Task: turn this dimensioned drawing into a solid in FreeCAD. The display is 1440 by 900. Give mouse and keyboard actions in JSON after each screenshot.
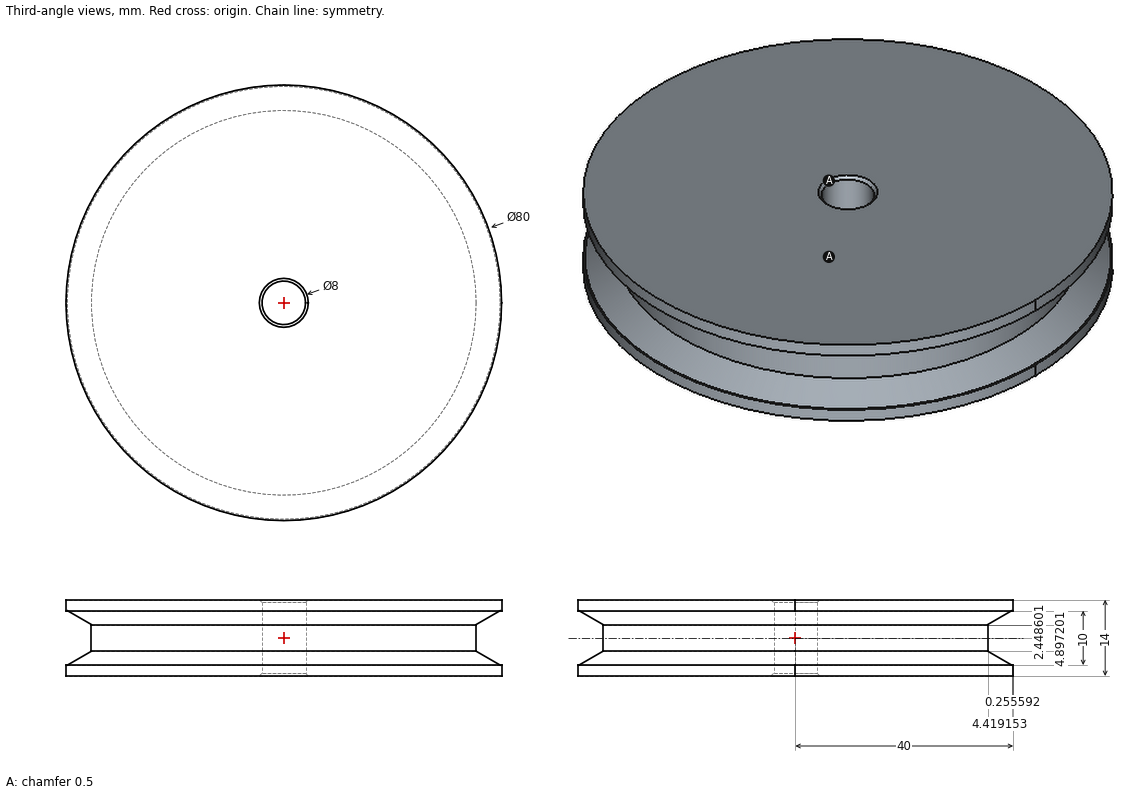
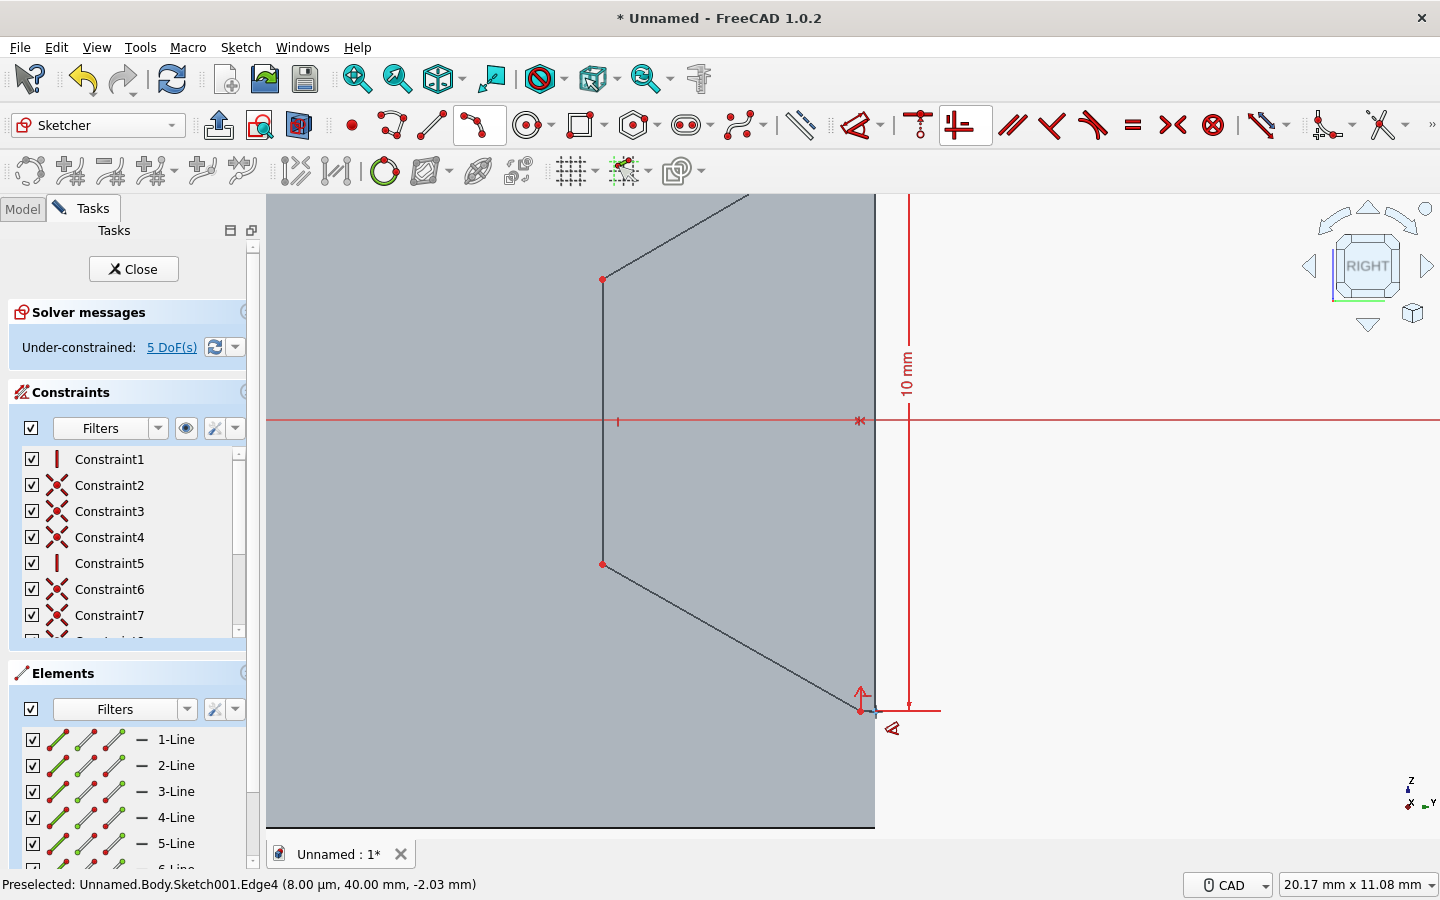
{"action": "left_click", "coordinate": [875, 711]}
{"action": "left_click", "coordinate": [585, 745]}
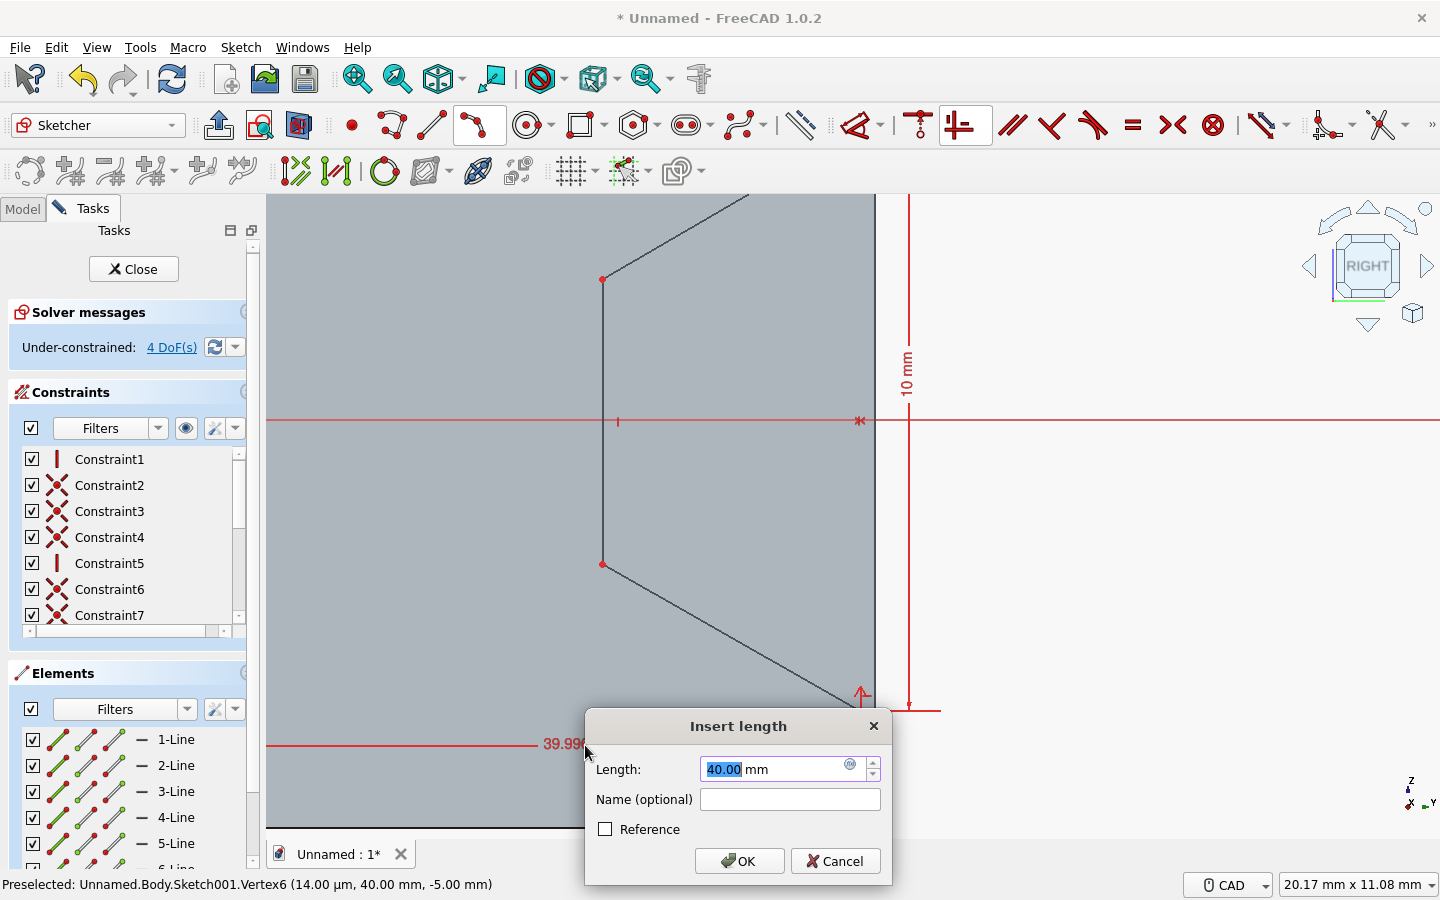
{"action": "type", "text": "40"}
{"action": "key", "text": "Return"}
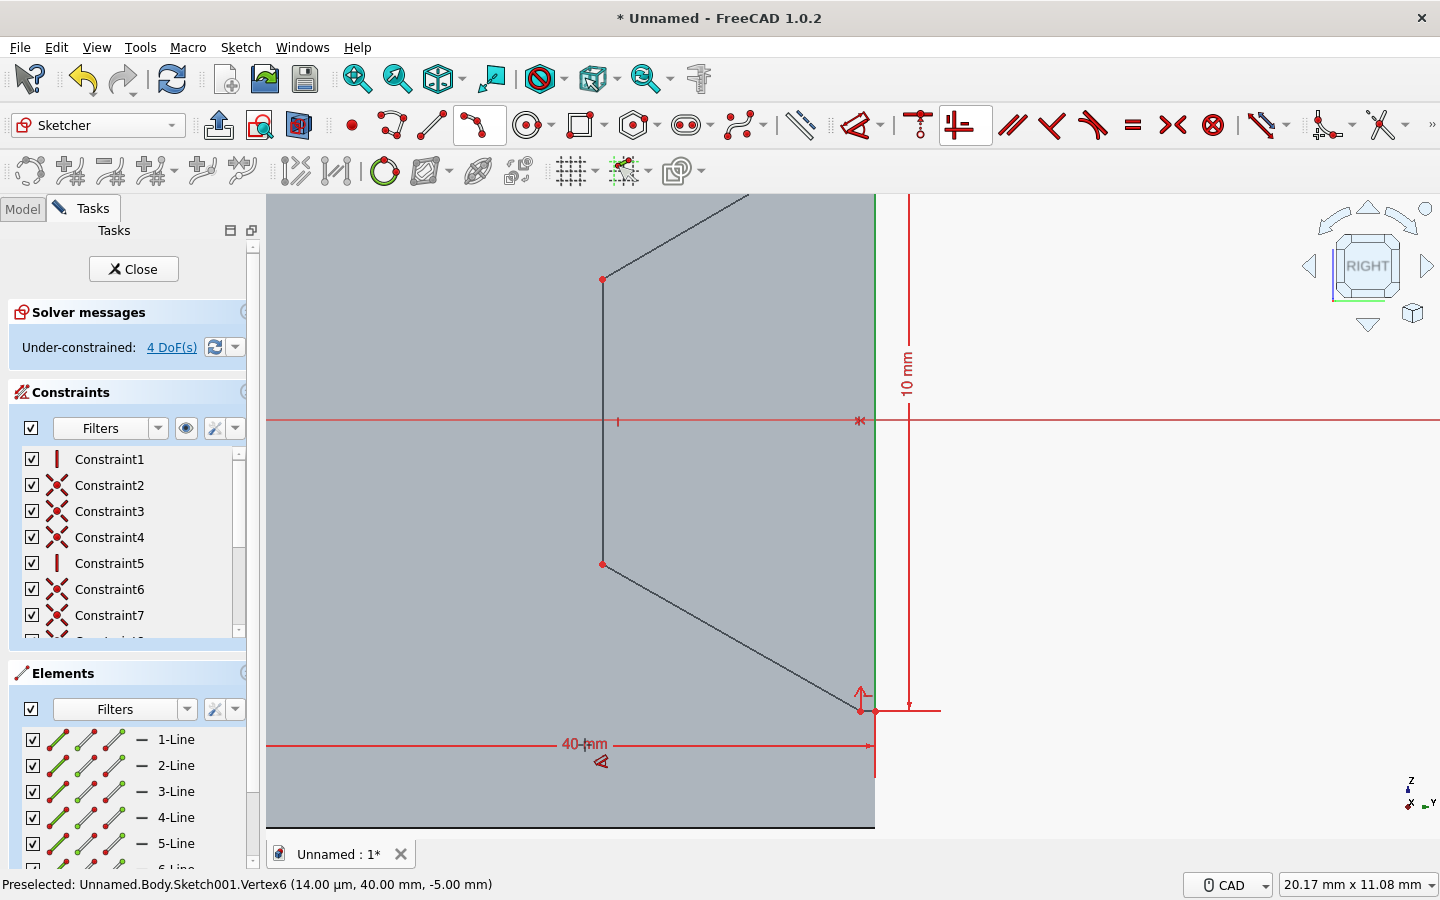
{"action": "left_click", "coordinate": [603, 365]}
{"action": "left_click", "coordinate": [569, 356]}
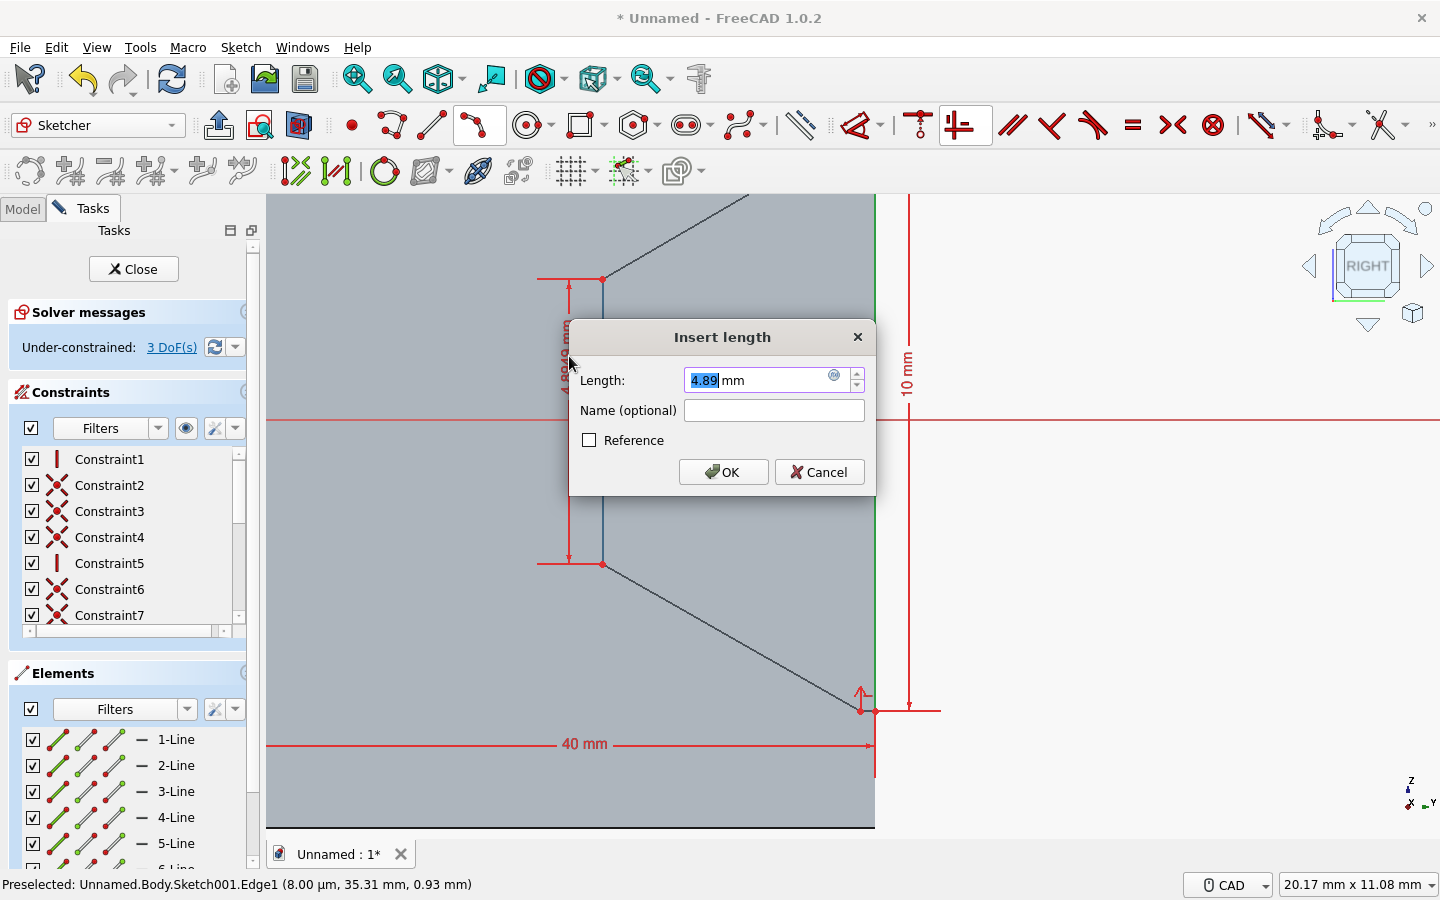
{"action": "type", "text": "4.897201"}
{"action": "key", "text": "Return"}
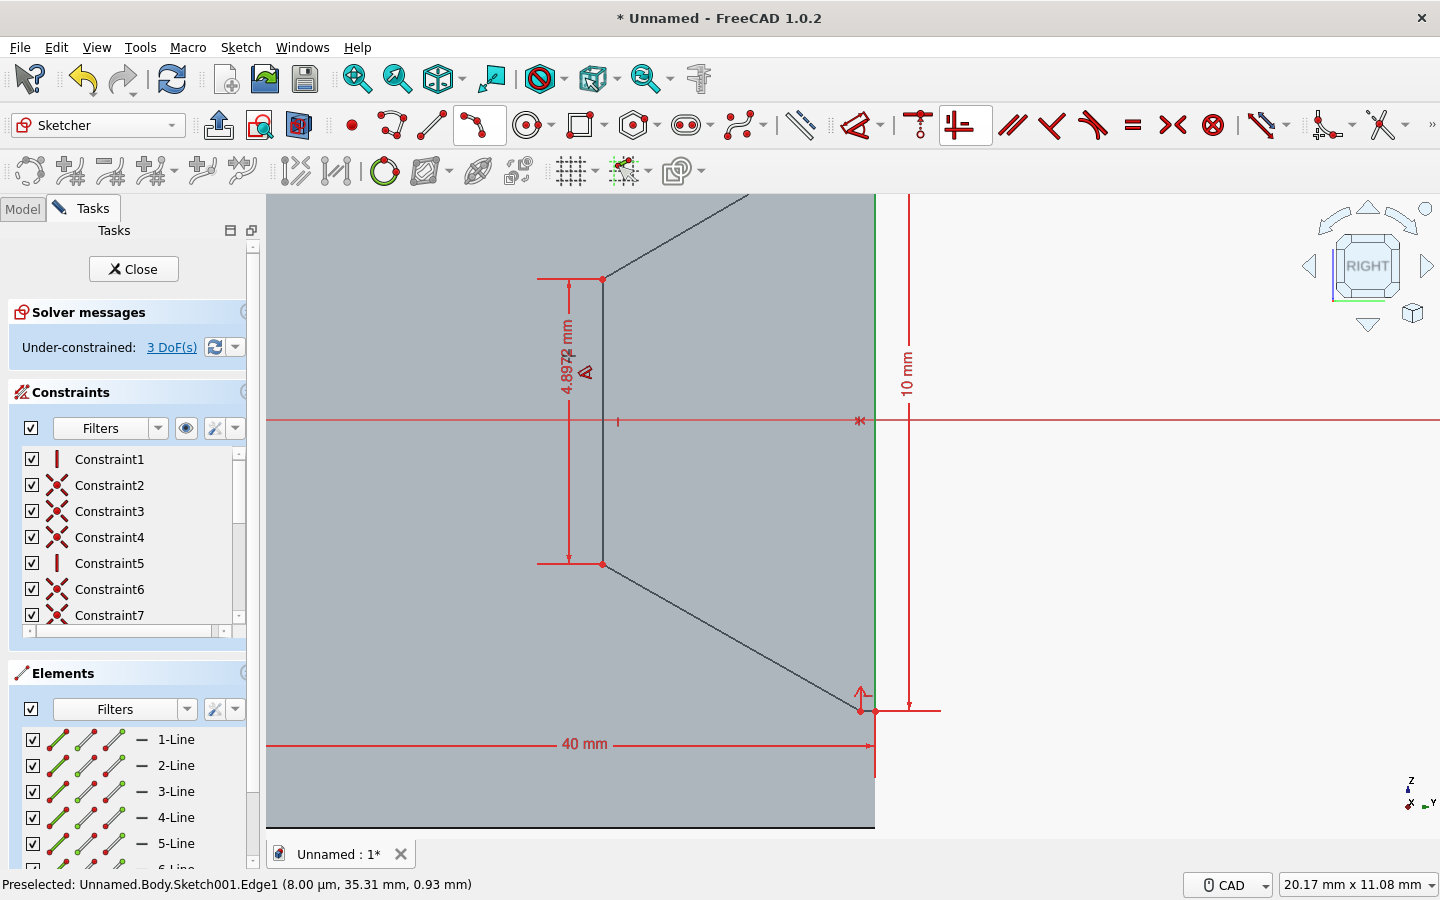
{"action": "scroll", "coordinate": [868, 711], "scroll_direction": "up", "scroll_amount": 5}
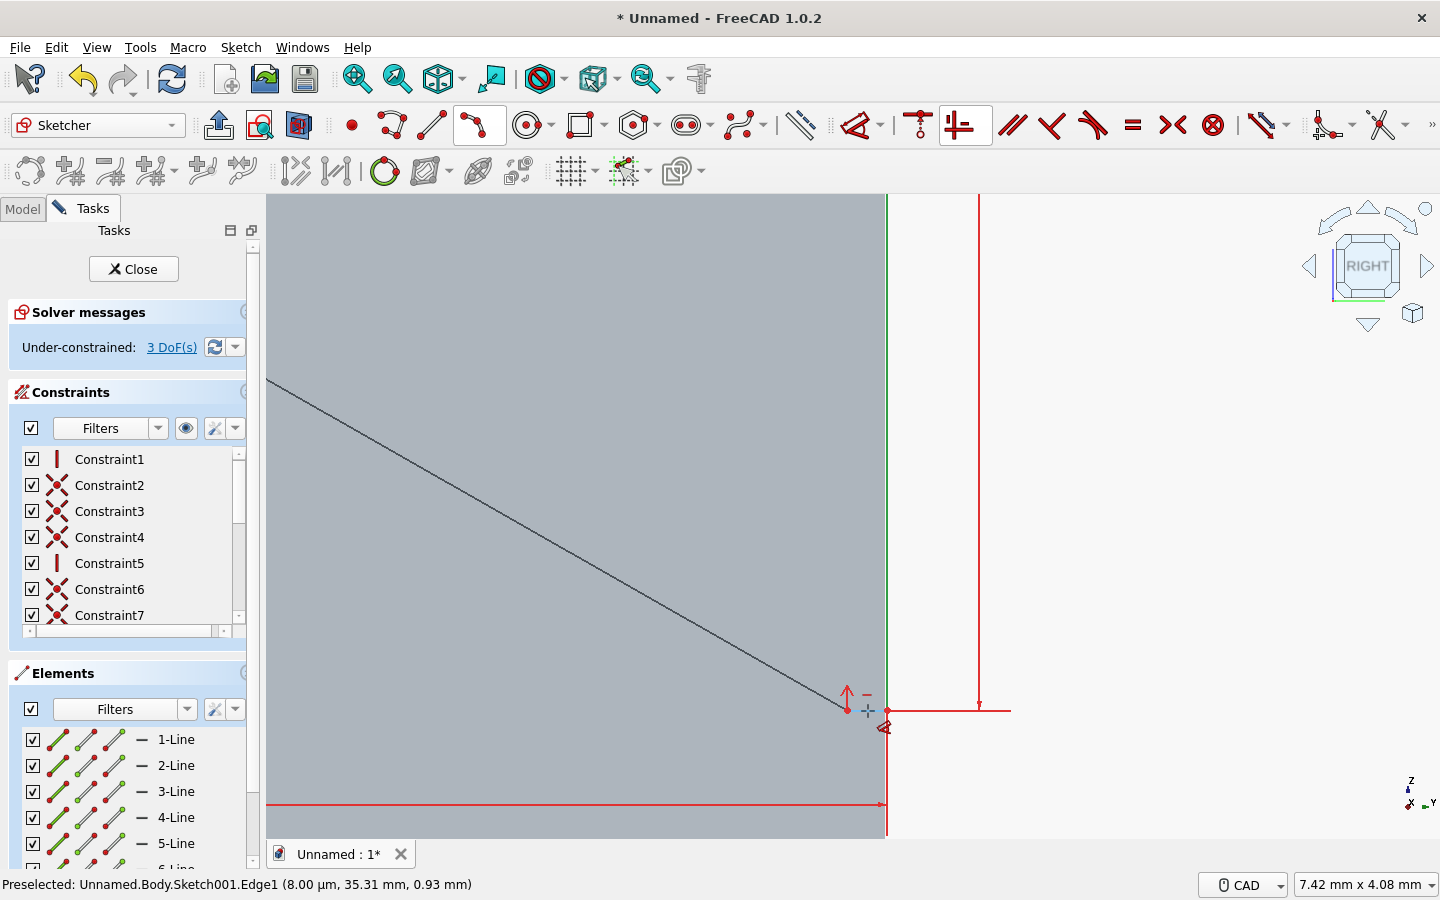
{"action": "left_click", "coordinate": [867, 711]}
{"action": "left_click", "coordinate": [867, 745]}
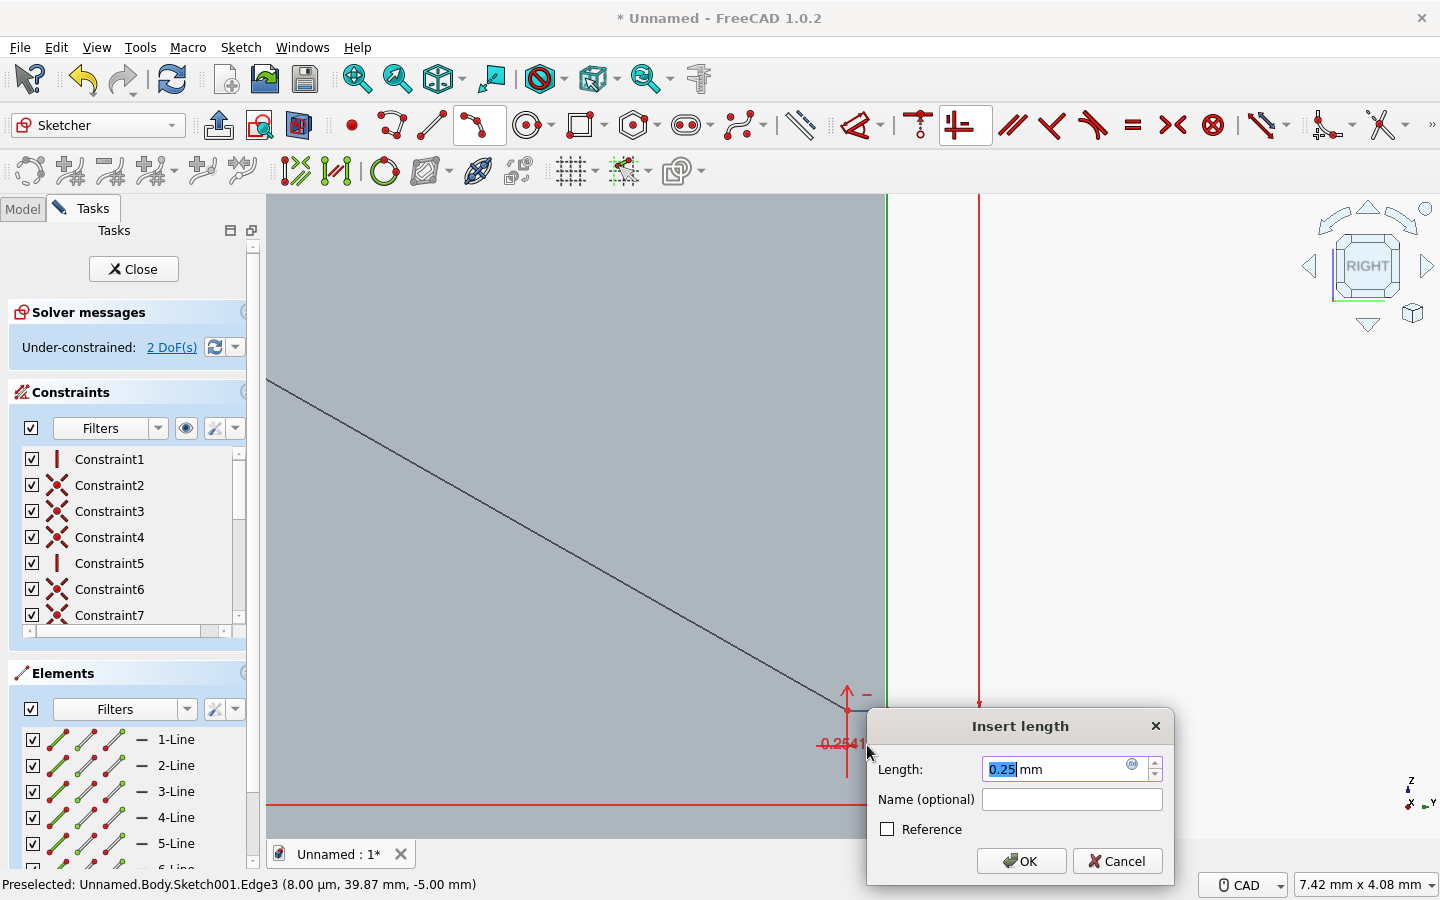
{"action": "type", "text": "0.255592"}
{"action": "key", "text": "Return"}